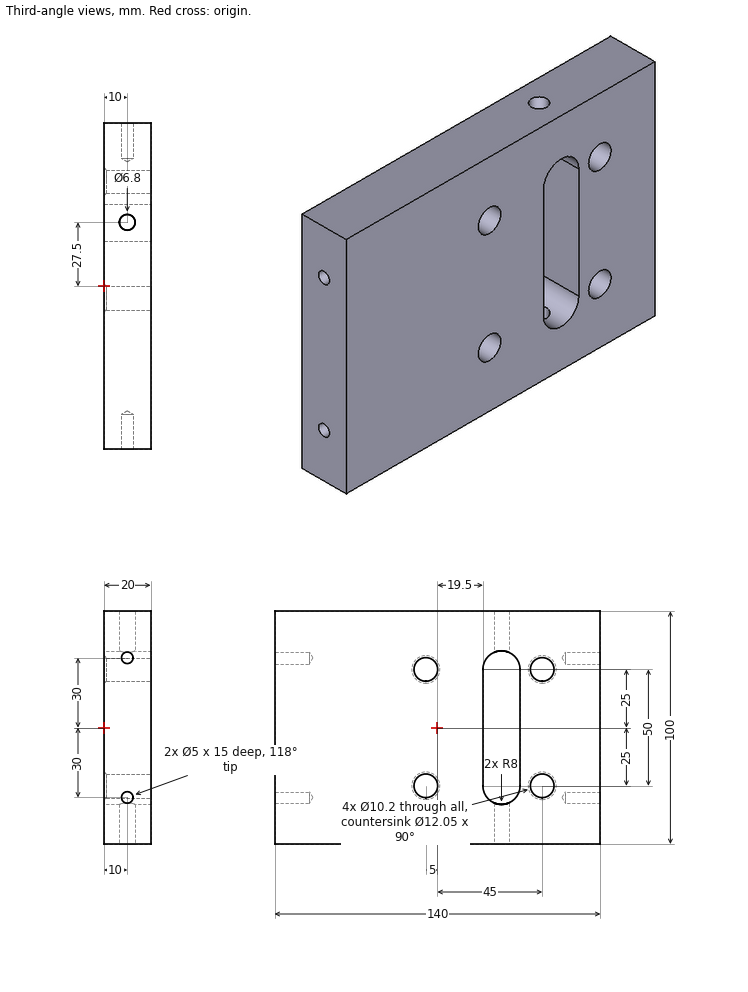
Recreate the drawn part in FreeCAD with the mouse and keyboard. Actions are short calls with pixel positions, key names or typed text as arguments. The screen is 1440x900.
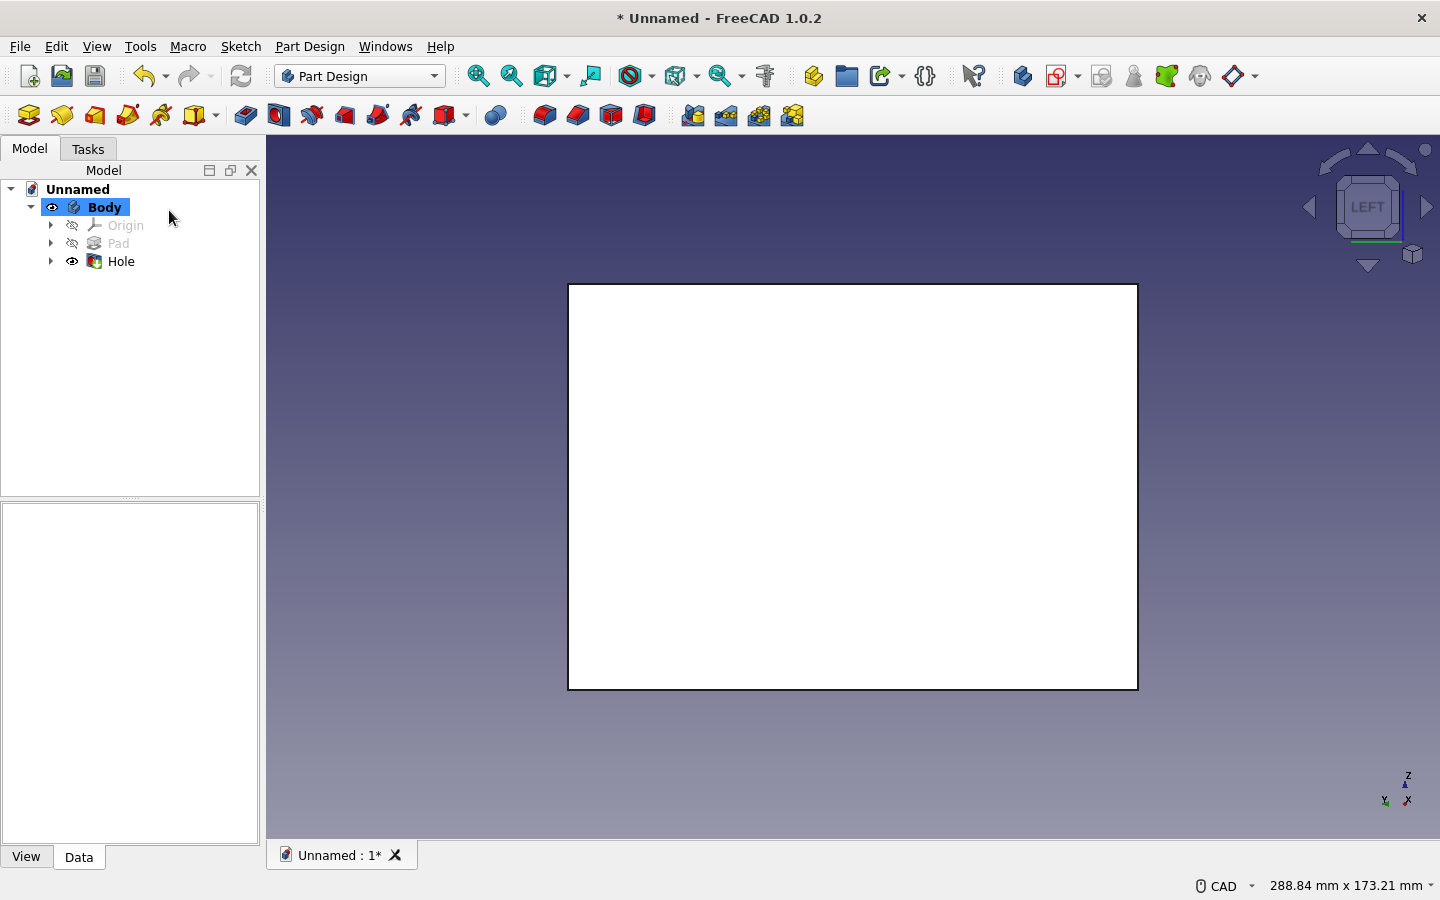
click(853, 486)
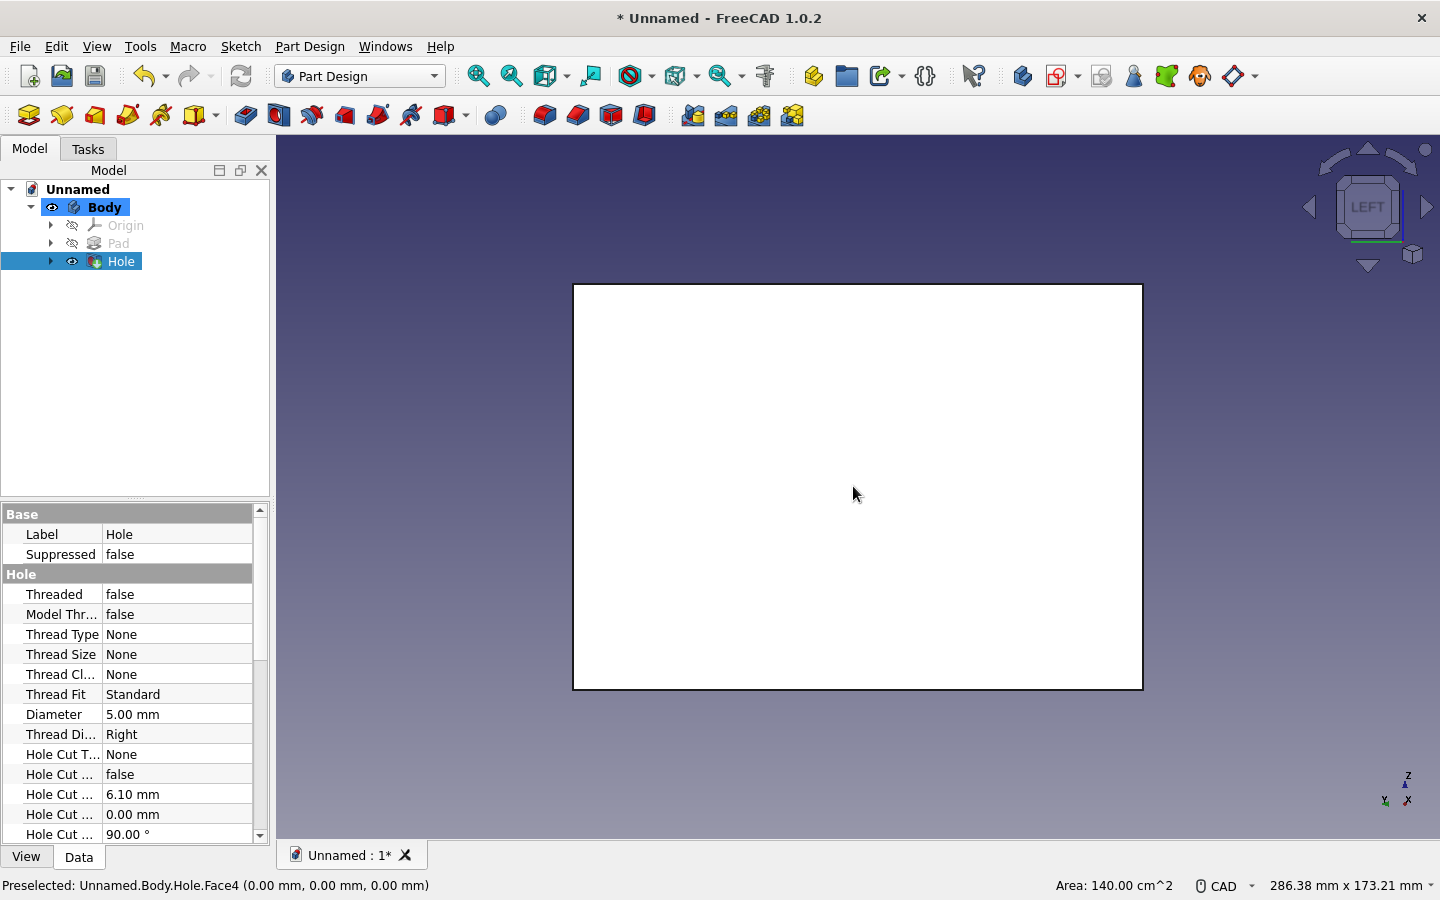
click(1056, 76)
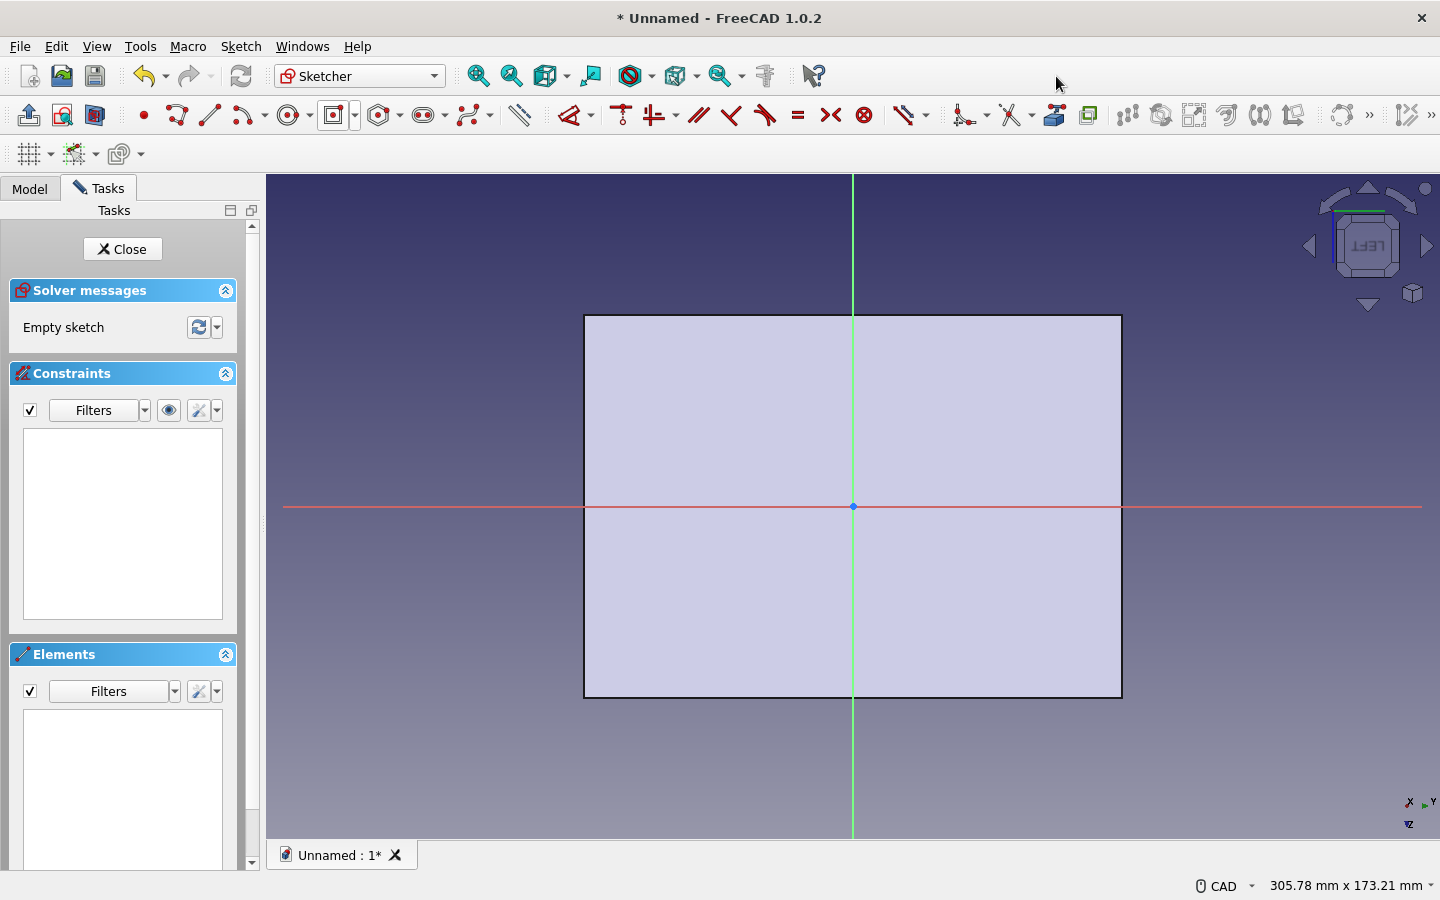
scroll(1087, 507, up, 3)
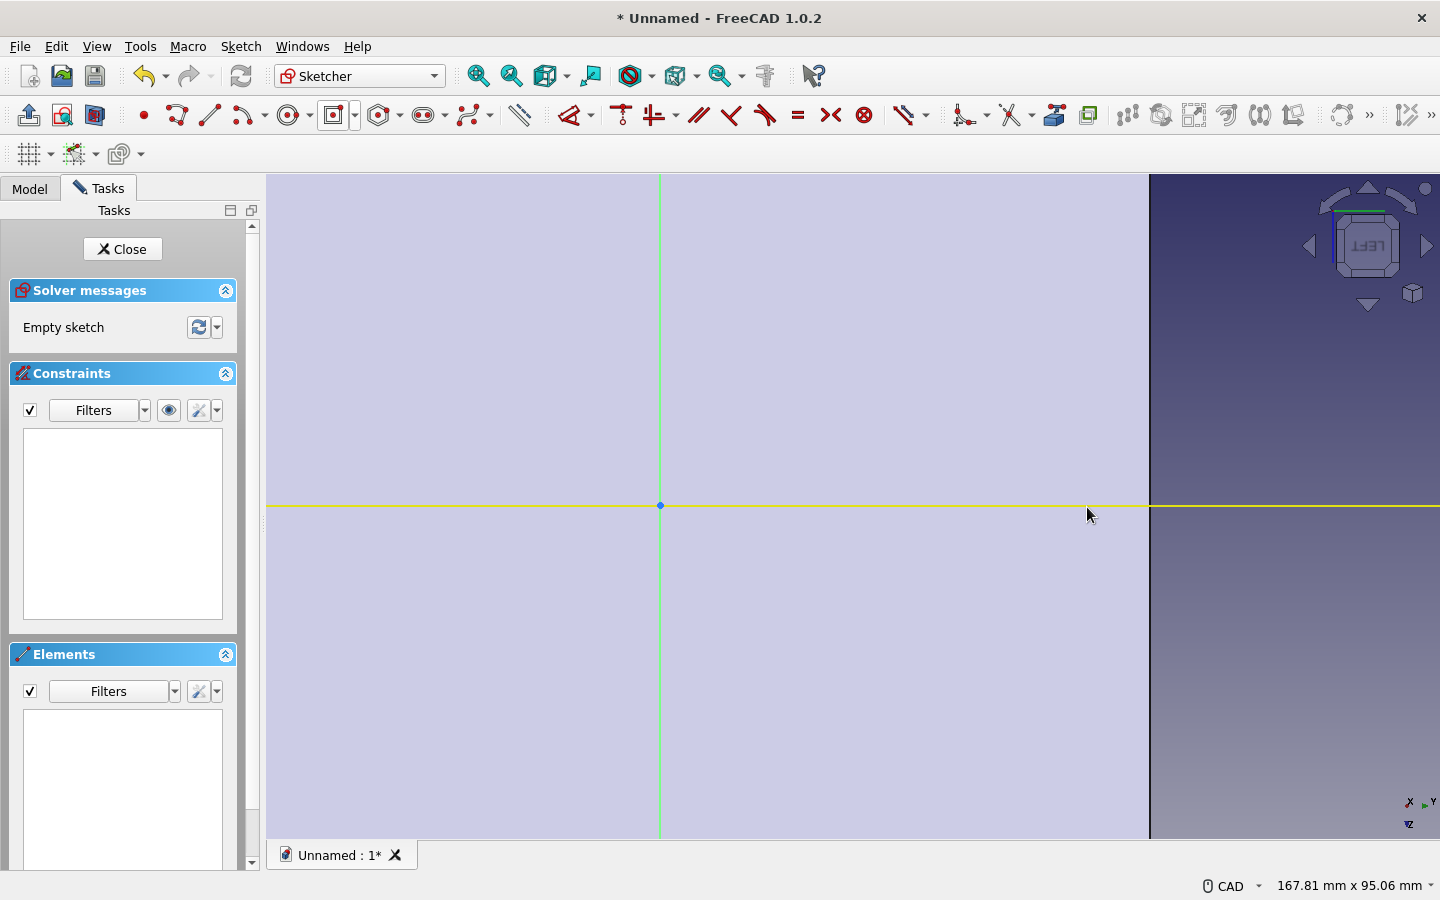
click(422, 116)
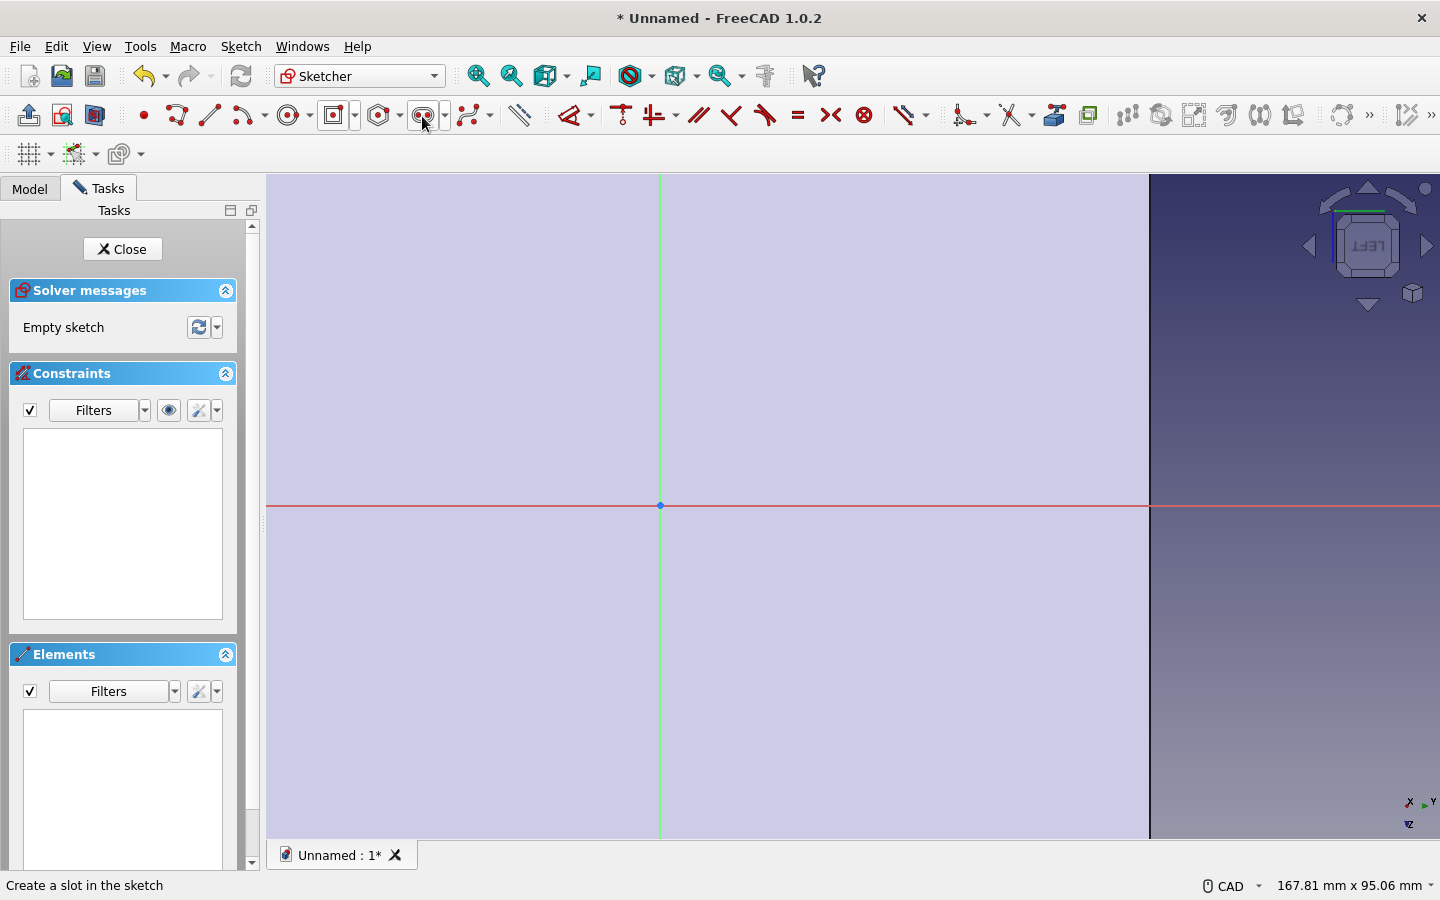
click(852, 681)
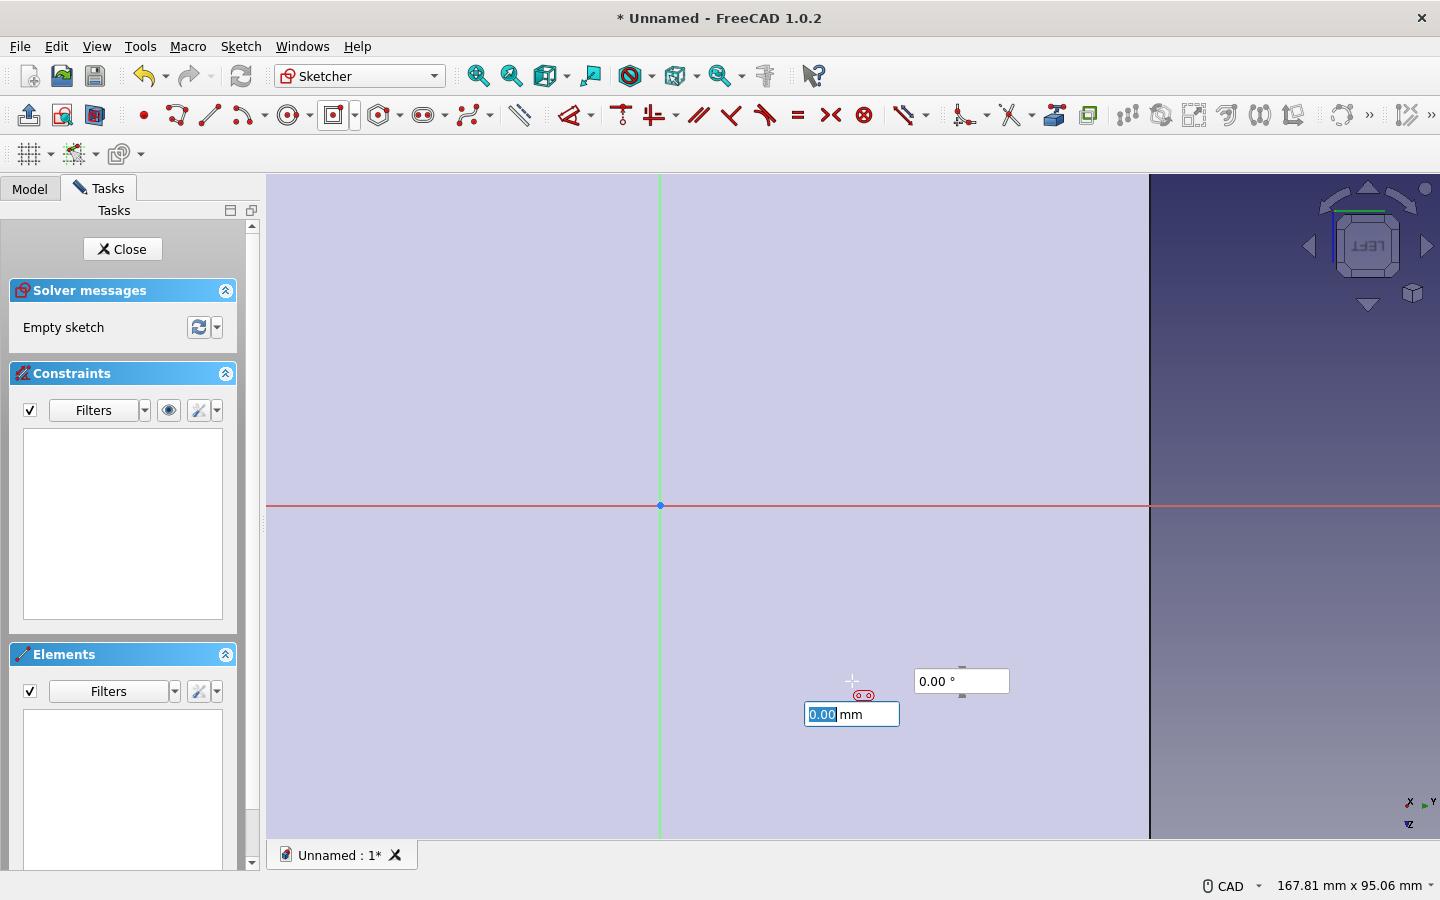
click(852, 331)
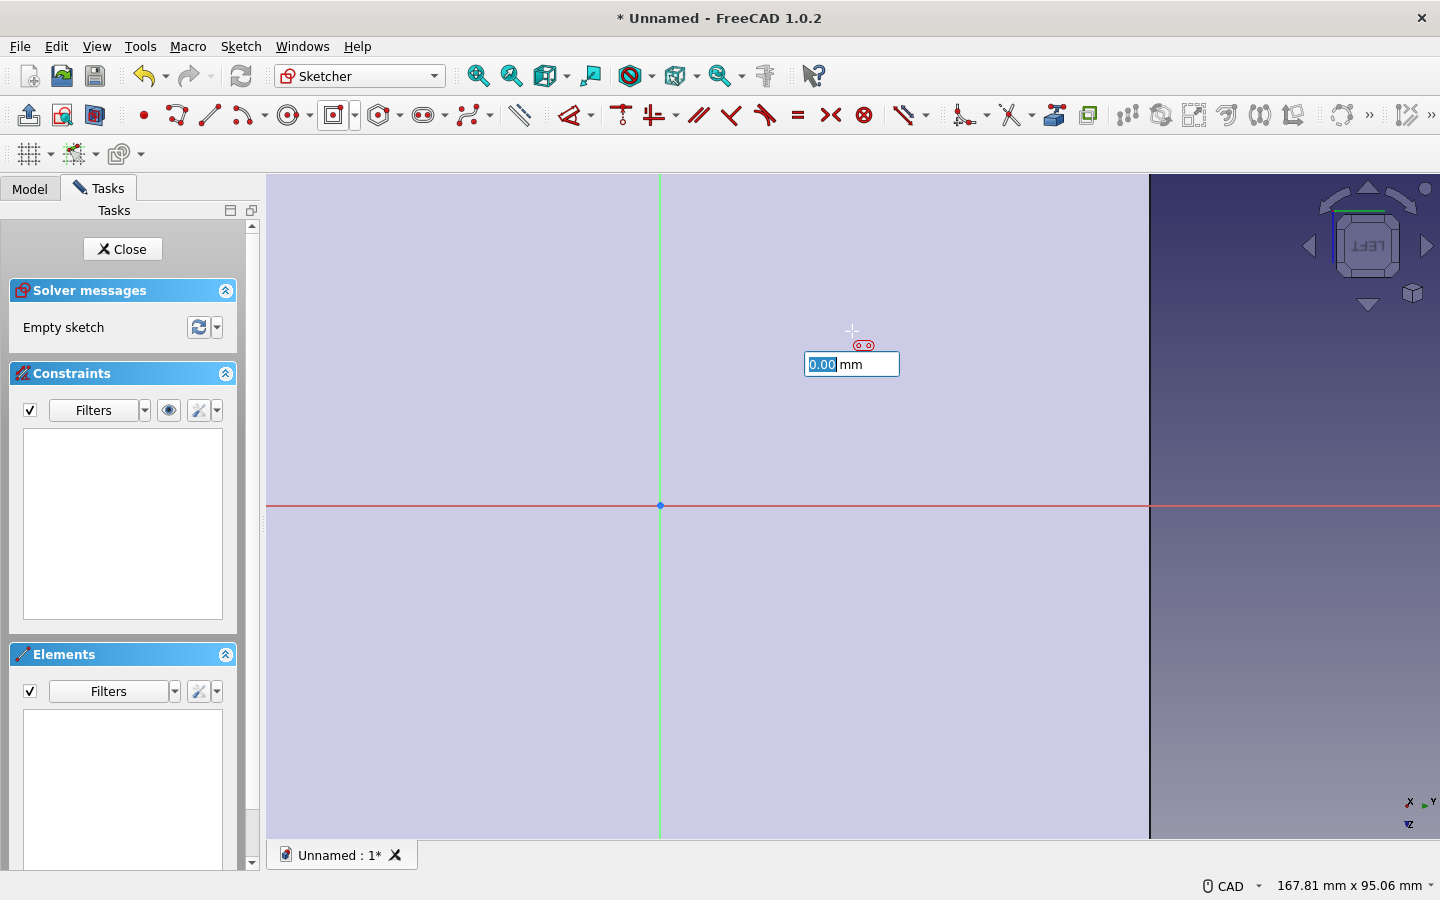
click(908, 558)
key(Escape)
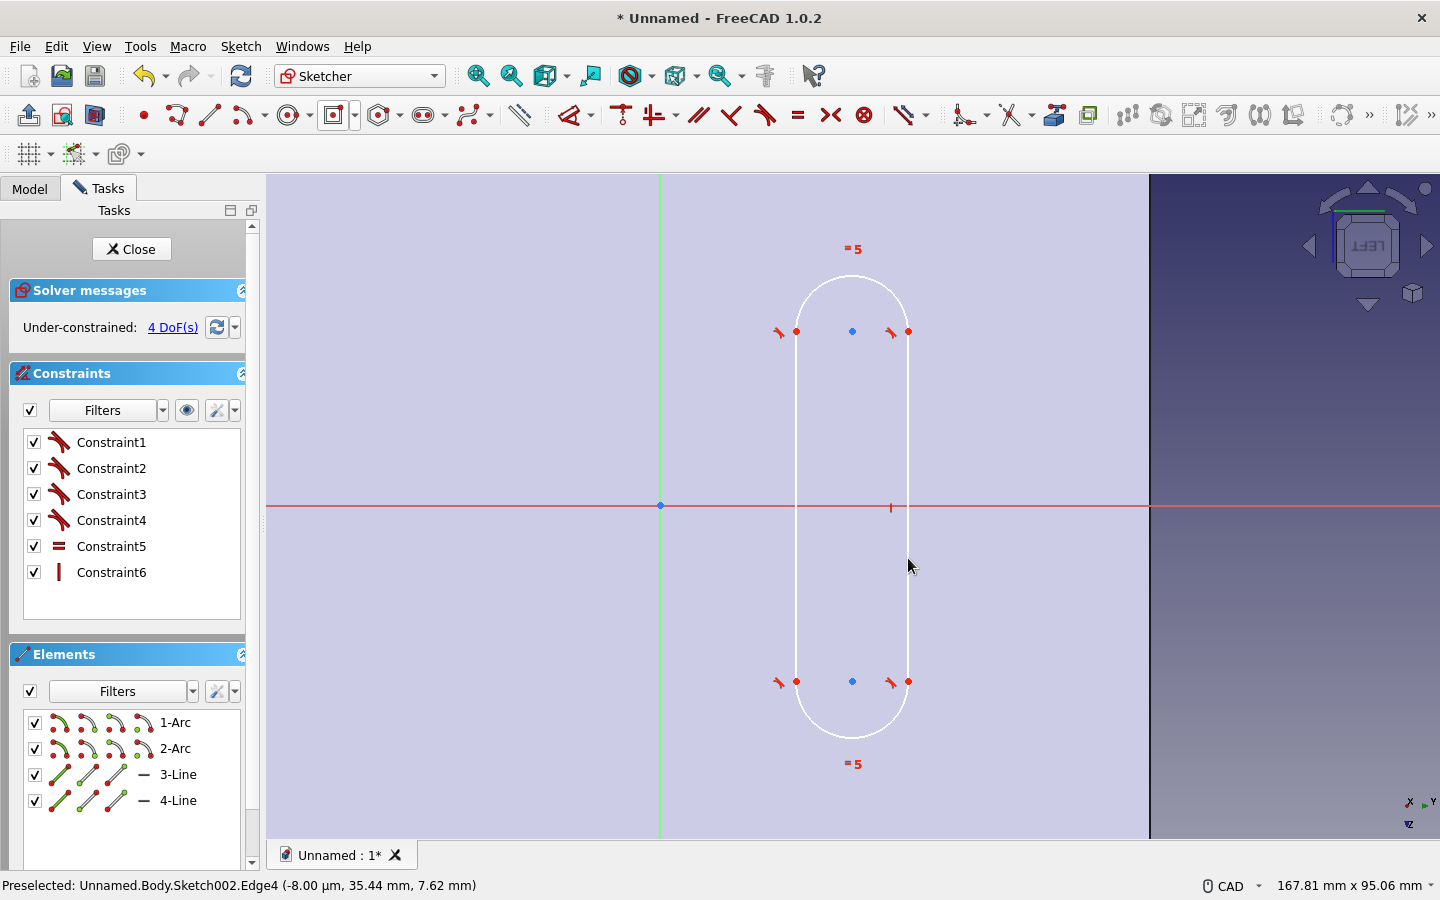
click(568, 116)